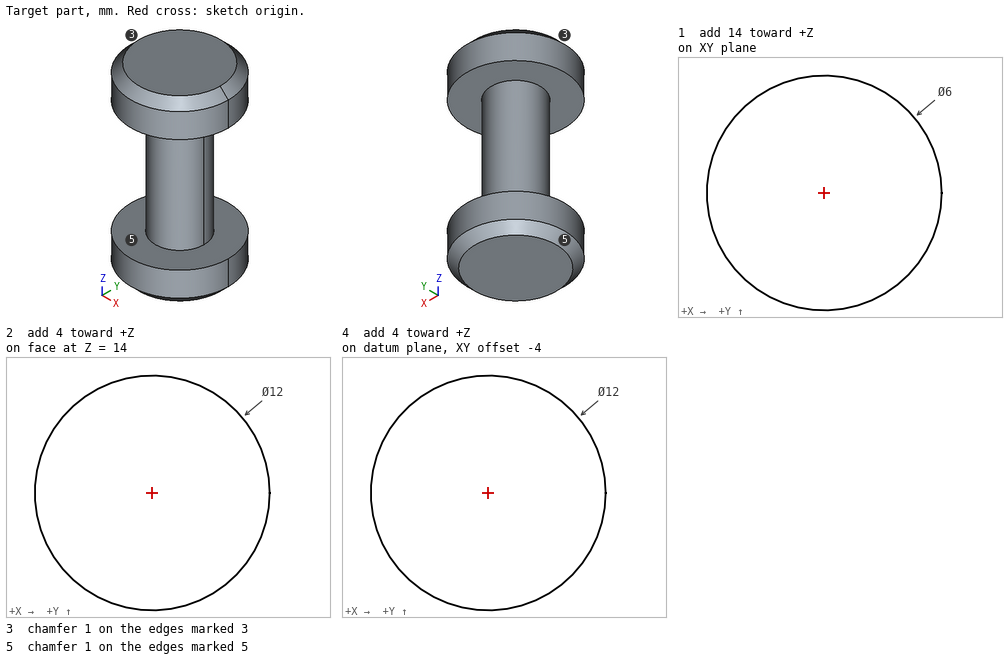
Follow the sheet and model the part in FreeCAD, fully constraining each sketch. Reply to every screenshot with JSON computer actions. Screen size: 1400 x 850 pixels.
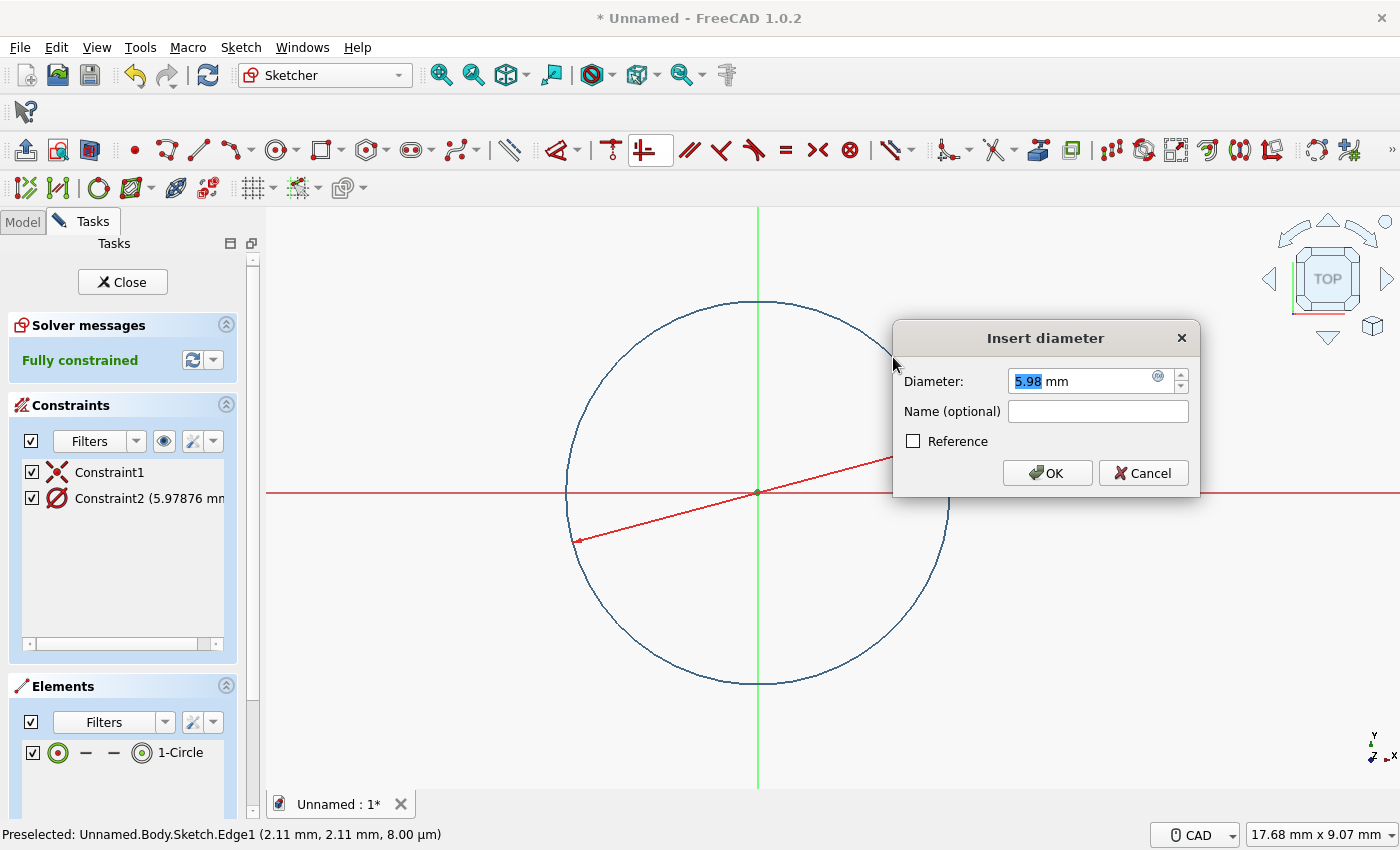
{"action": "type", "text": "6"}
{"action": "key", "text": "Return"}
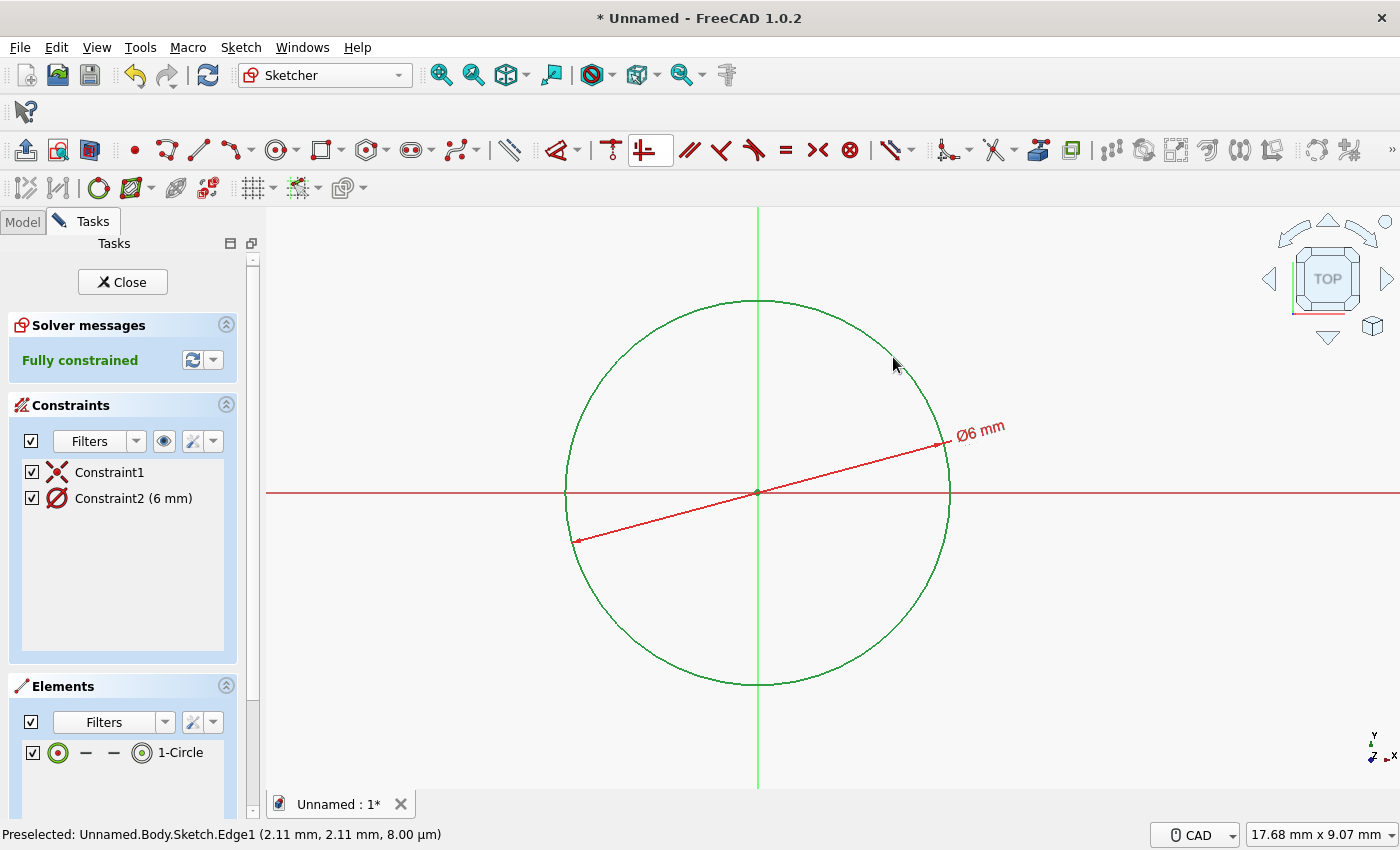
{"action": "left_click", "coordinate": [123, 282]}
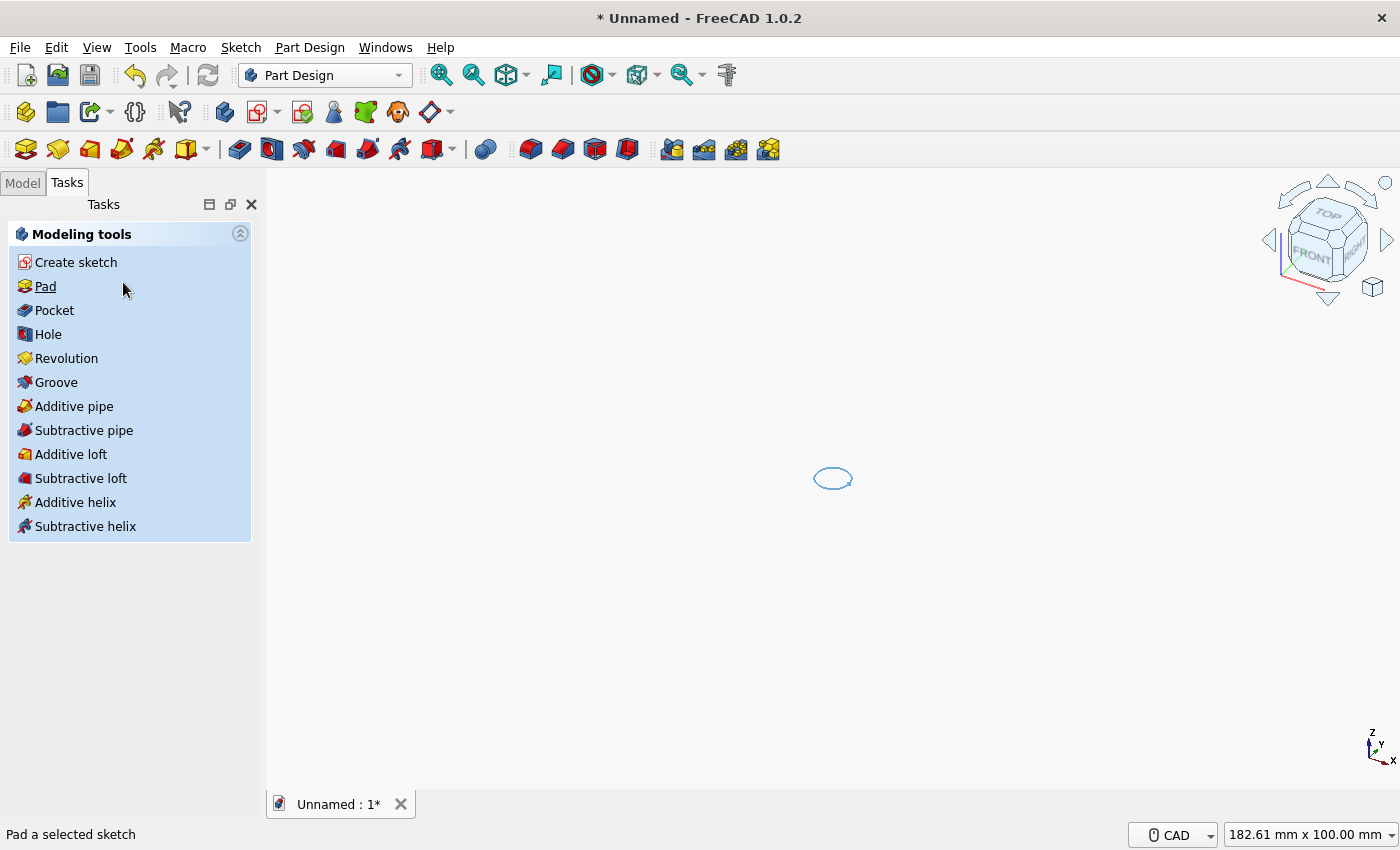
{"action": "left_click", "coordinate": [26, 150]}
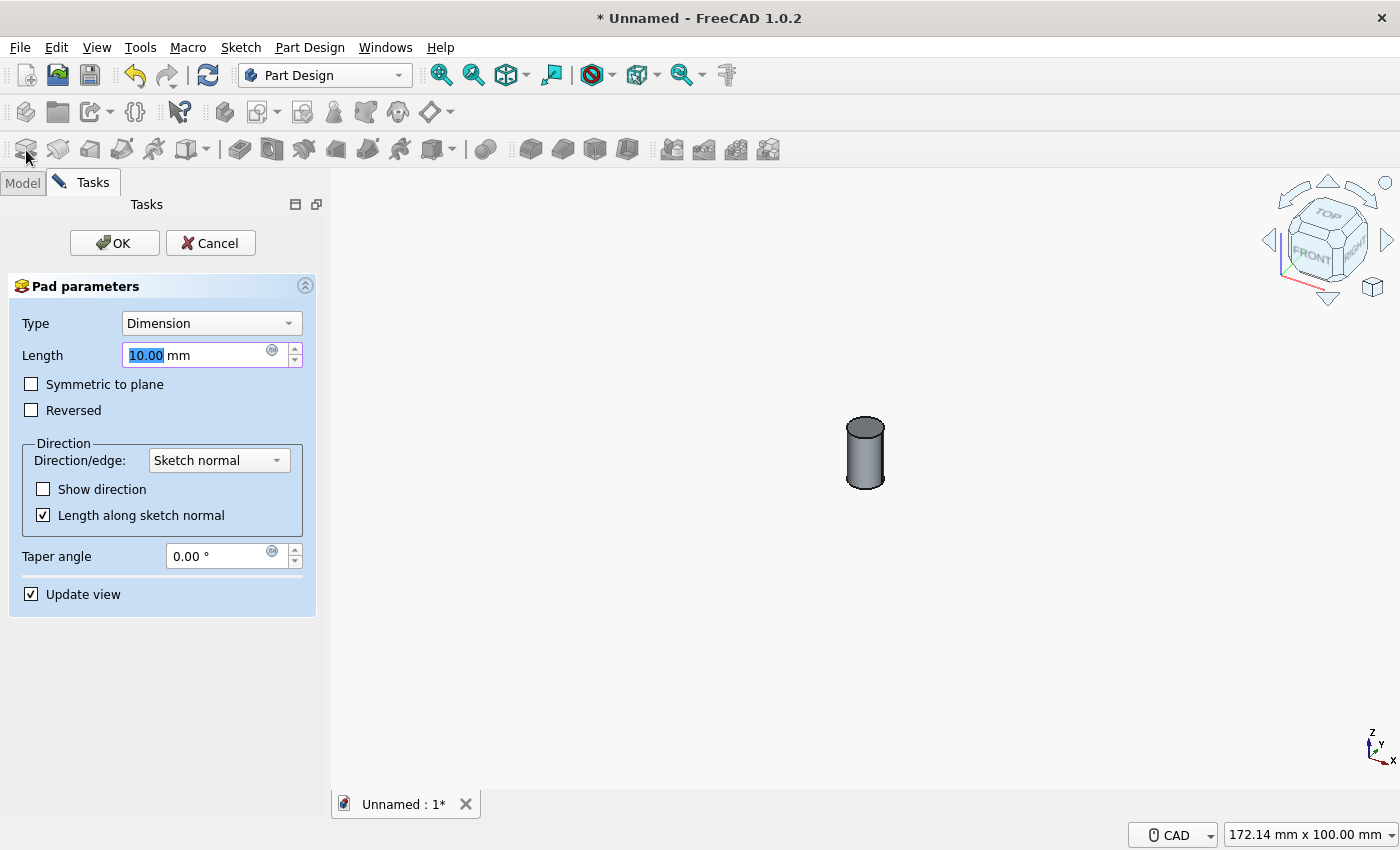
{"action": "type", "text": "14"}
{"action": "key", "text": "Tab"}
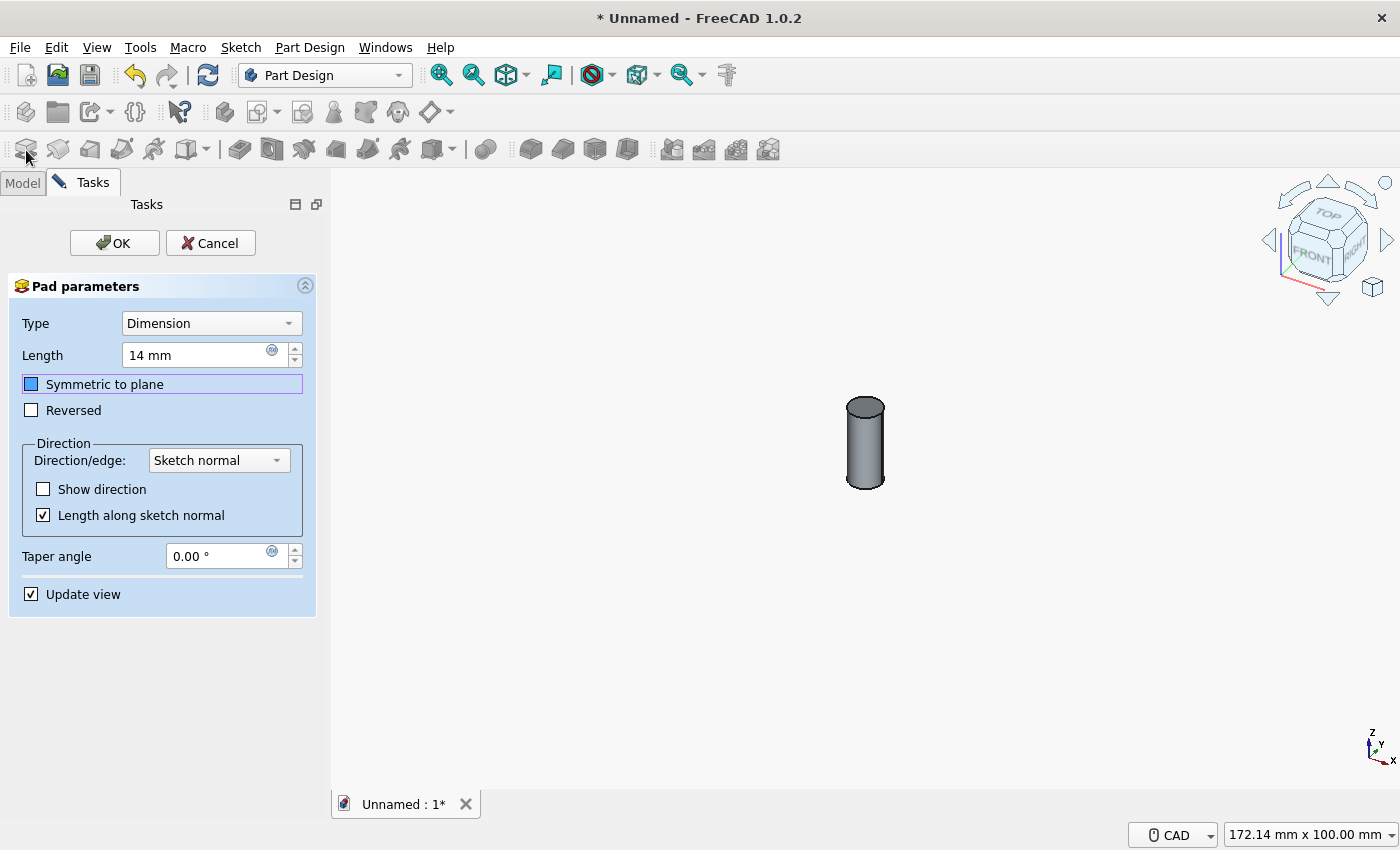
{"action": "left_click", "coordinate": [115, 243]}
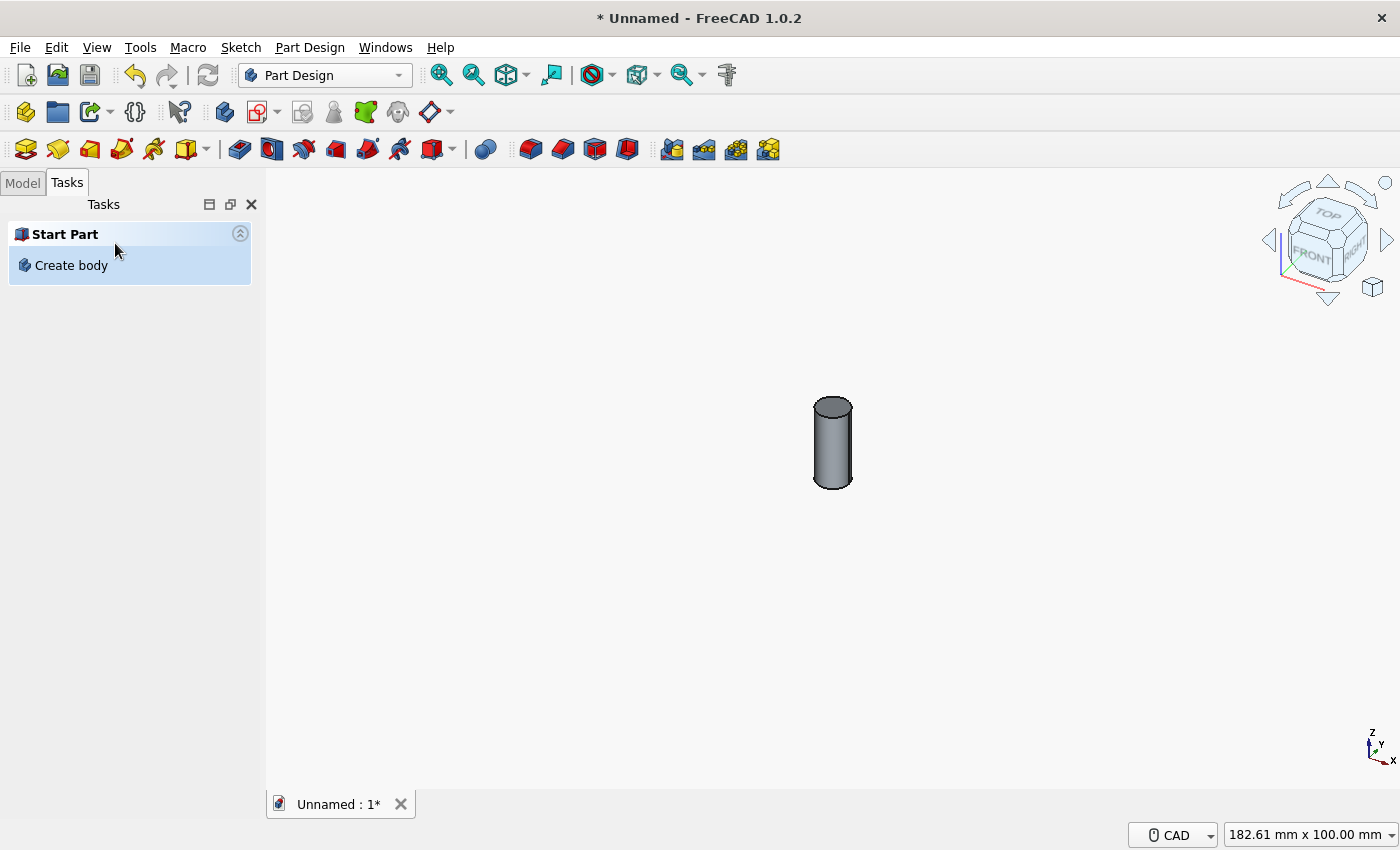
{"action": "left_click", "coordinate": [442, 76]}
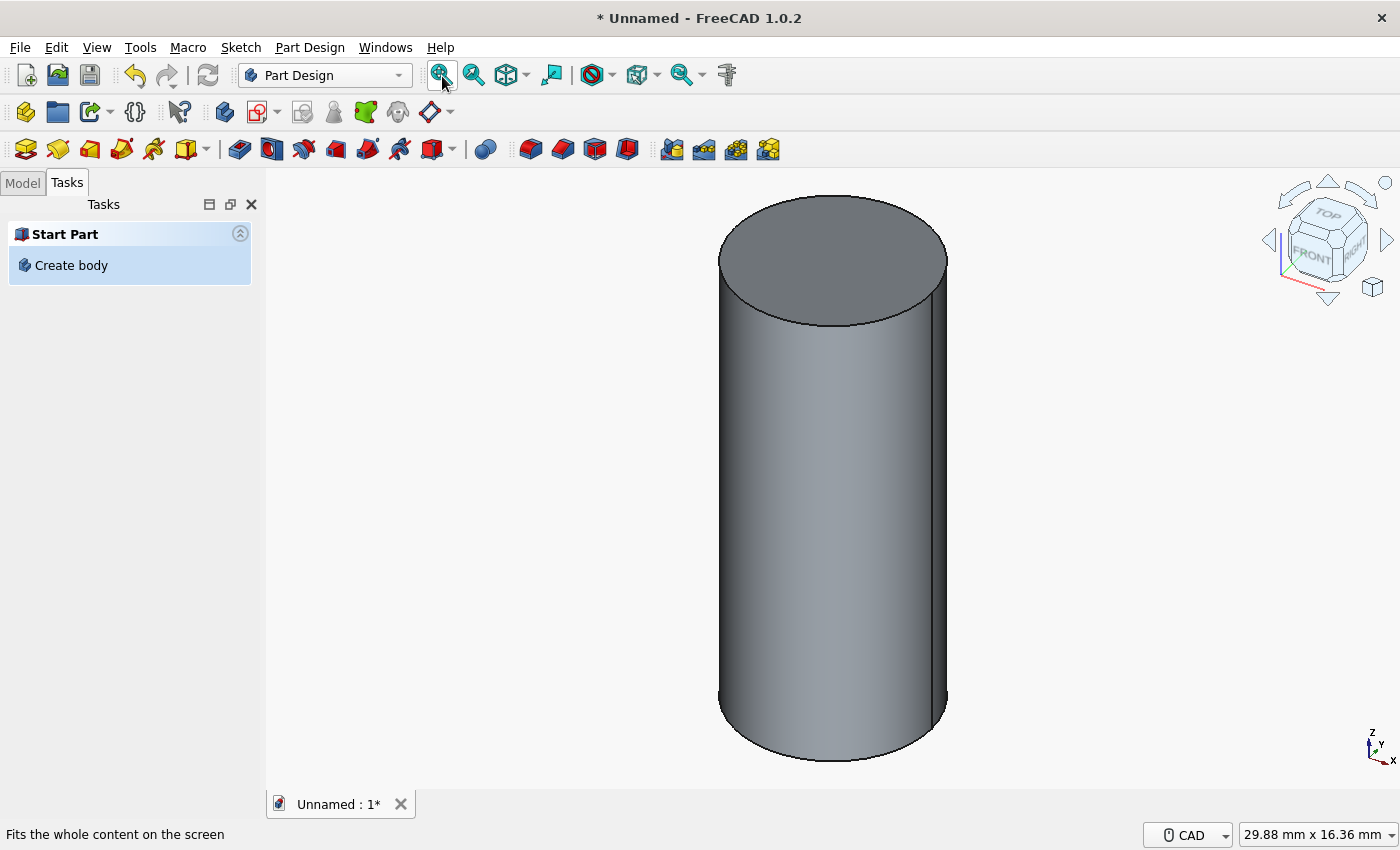
{"action": "left_click", "coordinate": [833, 260]}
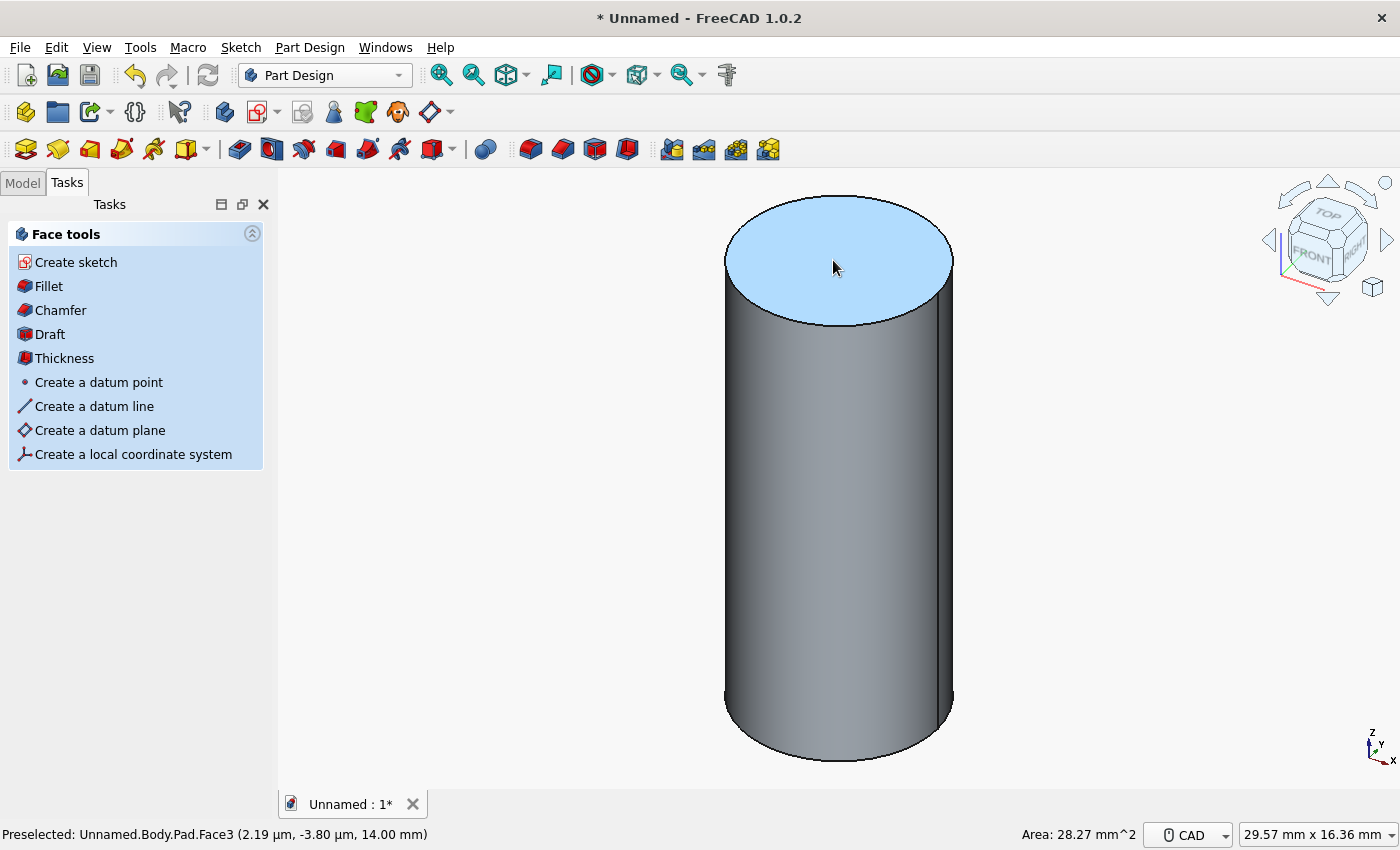
{"action": "left_click", "coordinate": [258, 112]}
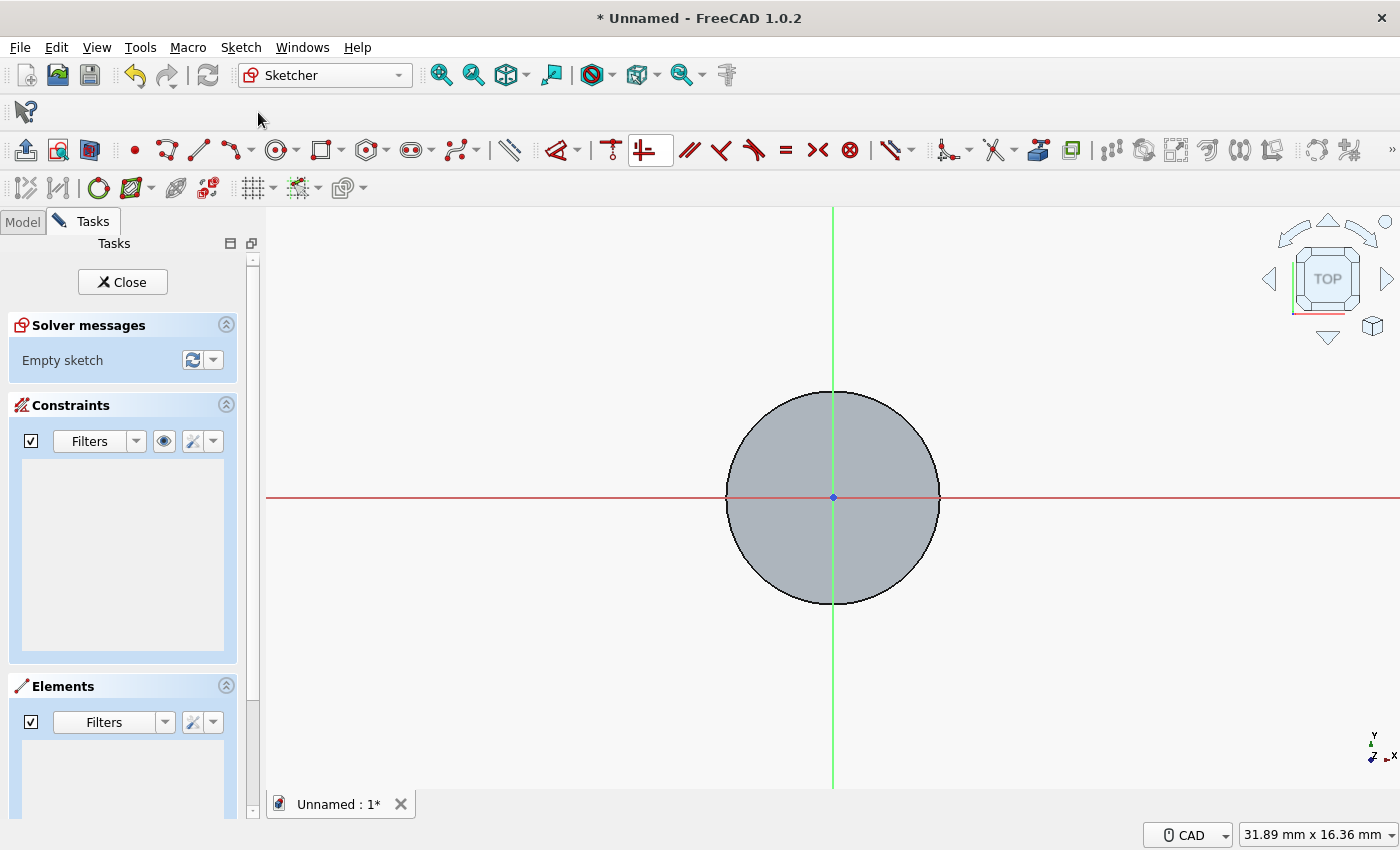
{"action": "key", "text": "g c"}